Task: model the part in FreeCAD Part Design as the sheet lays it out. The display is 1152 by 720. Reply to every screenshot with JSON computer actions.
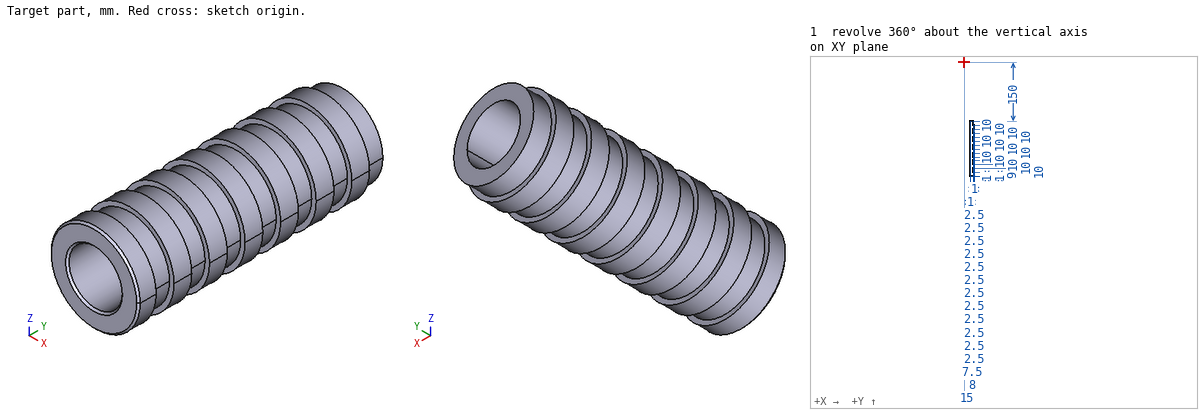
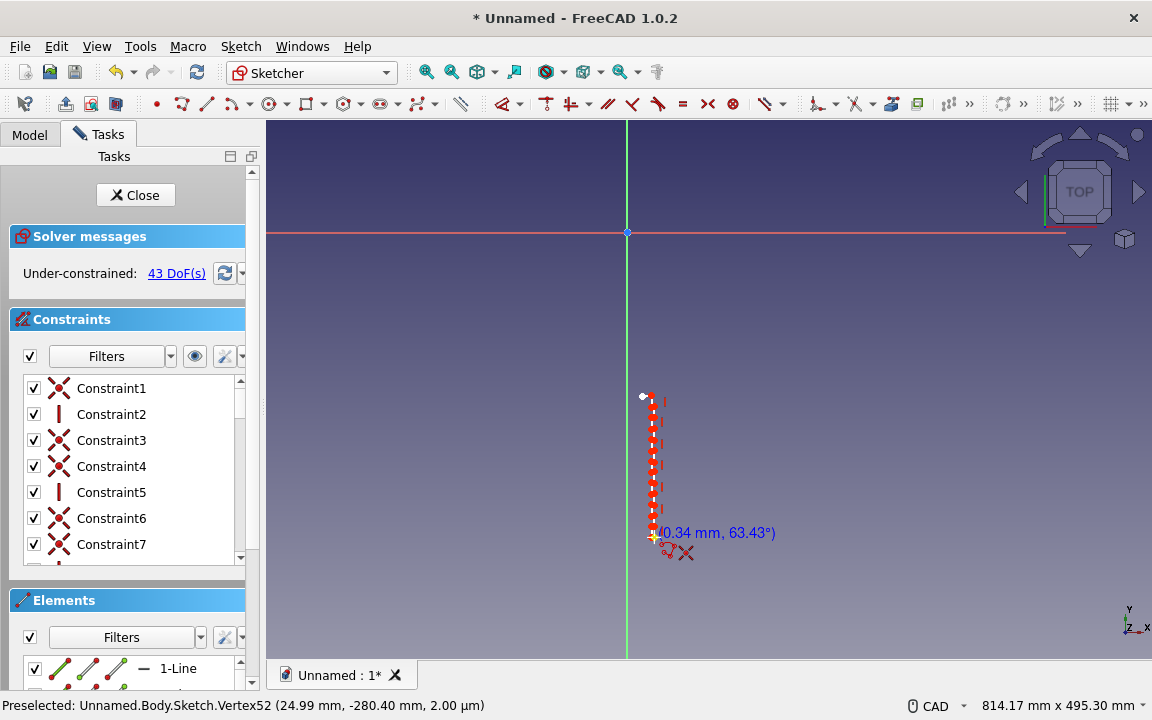
{"action": "scroll", "coordinate": [654, 547], "scroll_direction": "up", "scroll_amount": 3}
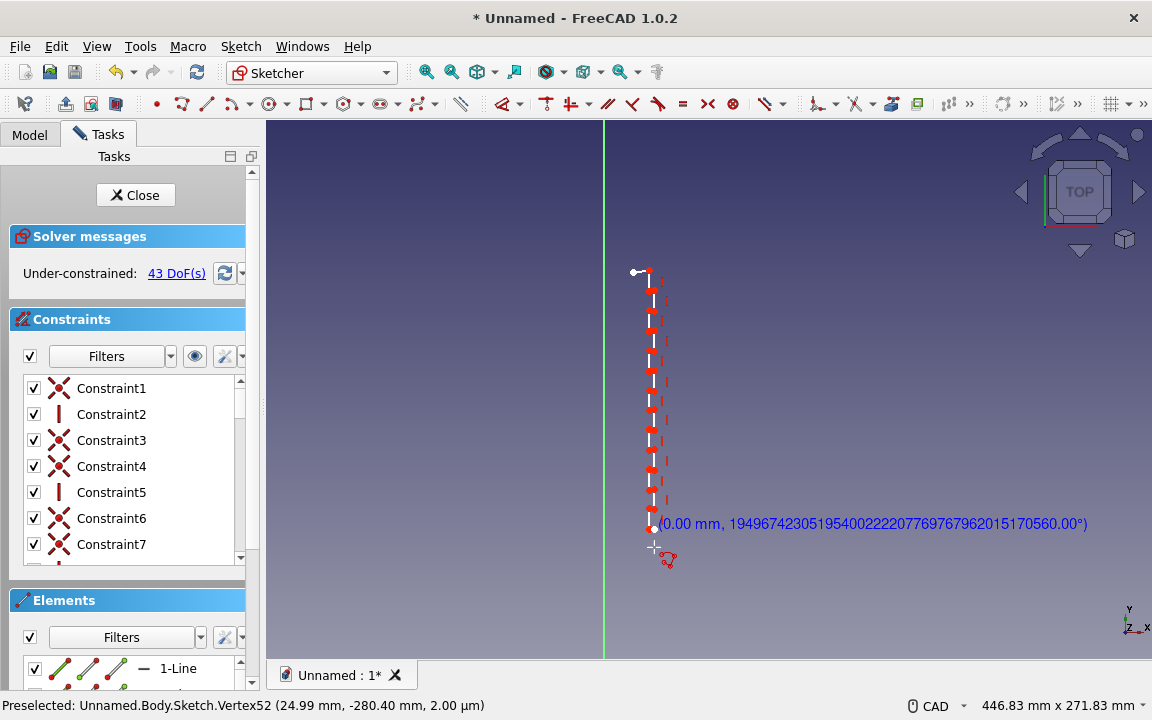
{"action": "left_click", "coordinate": [654, 546]}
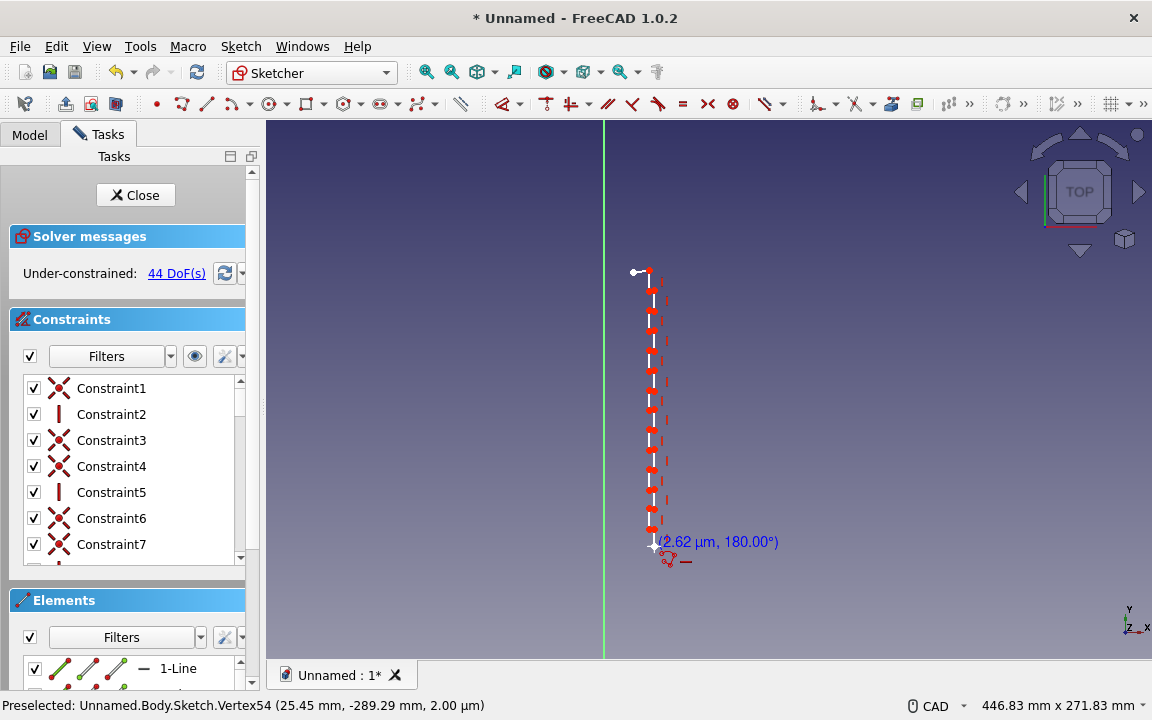
{"action": "scroll", "coordinate": [652, 548], "scroll_direction": "up", "scroll_amount": 9}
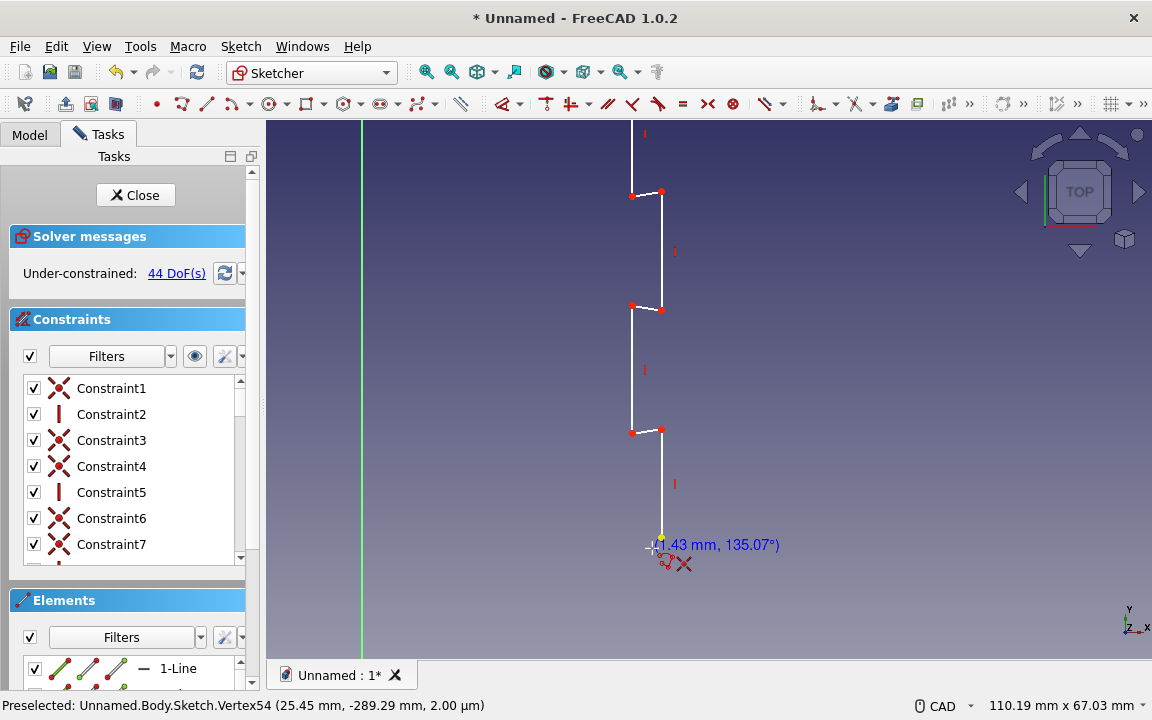
{"action": "left_click", "coordinate": [650, 546]}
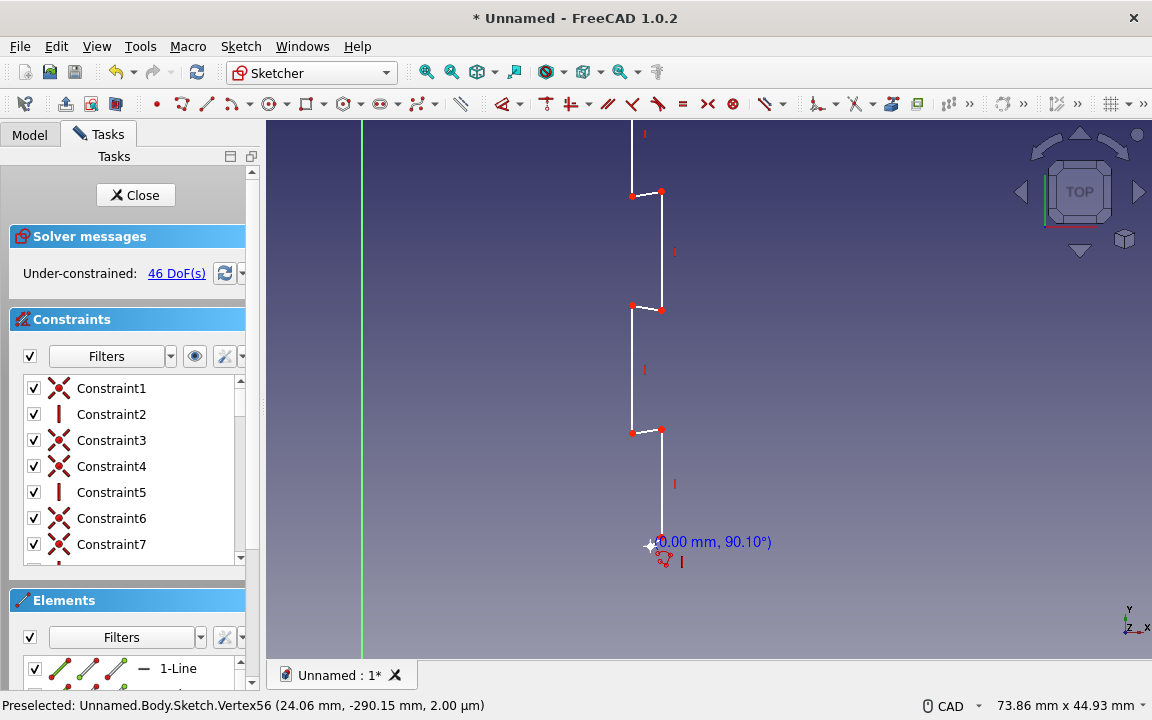
{"action": "scroll", "coordinate": [653, 547], "scroll_direction": "down", "scroll_amount": 12}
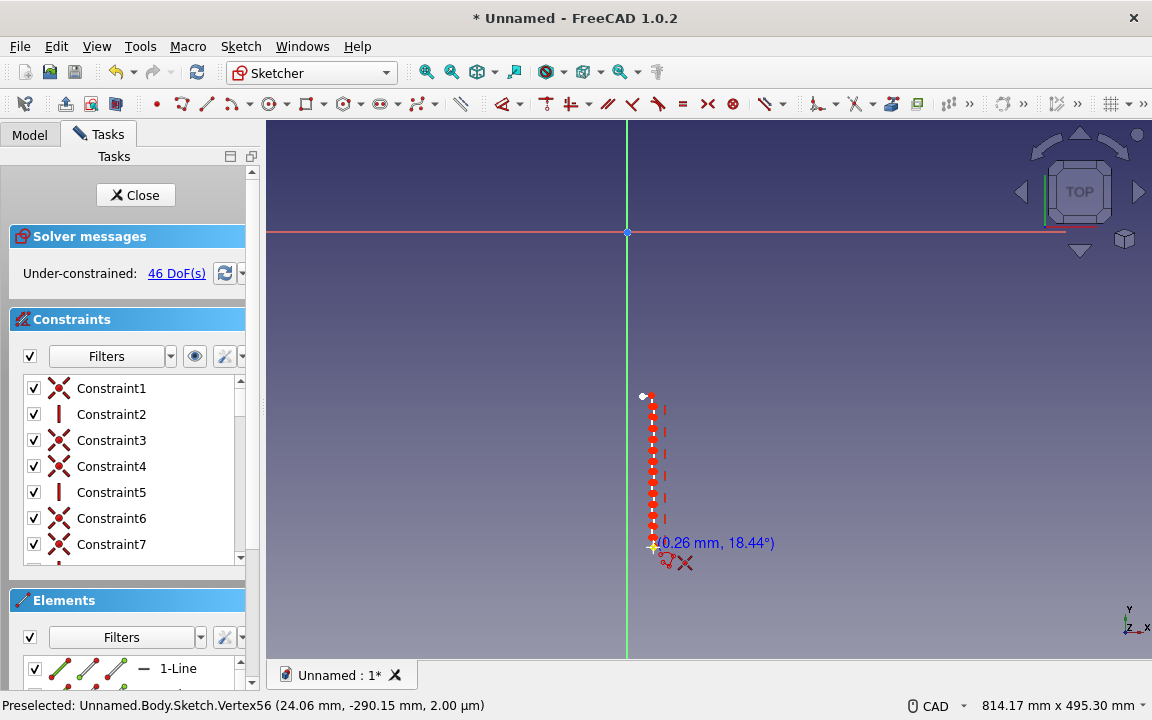
{"action": "scroll", "coordinate": [644, 548], "scroll_direction": "up", "scroll_amount": 4}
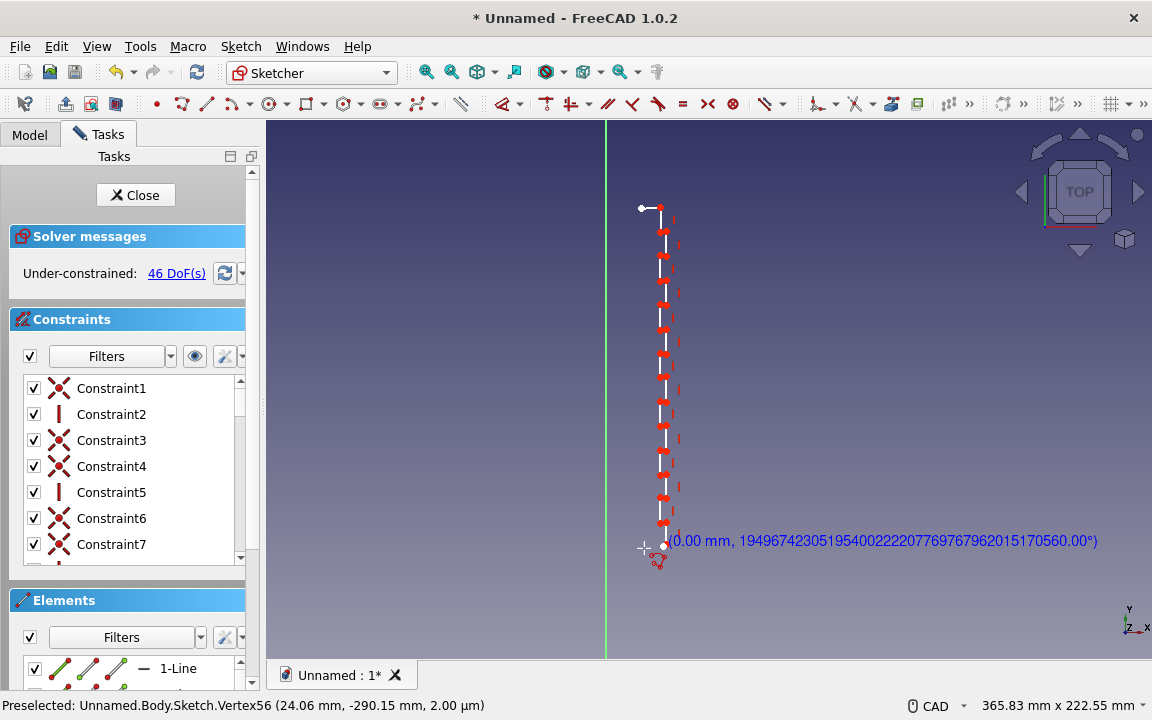
{"action": "left_click", "coordinate": [644, 546]}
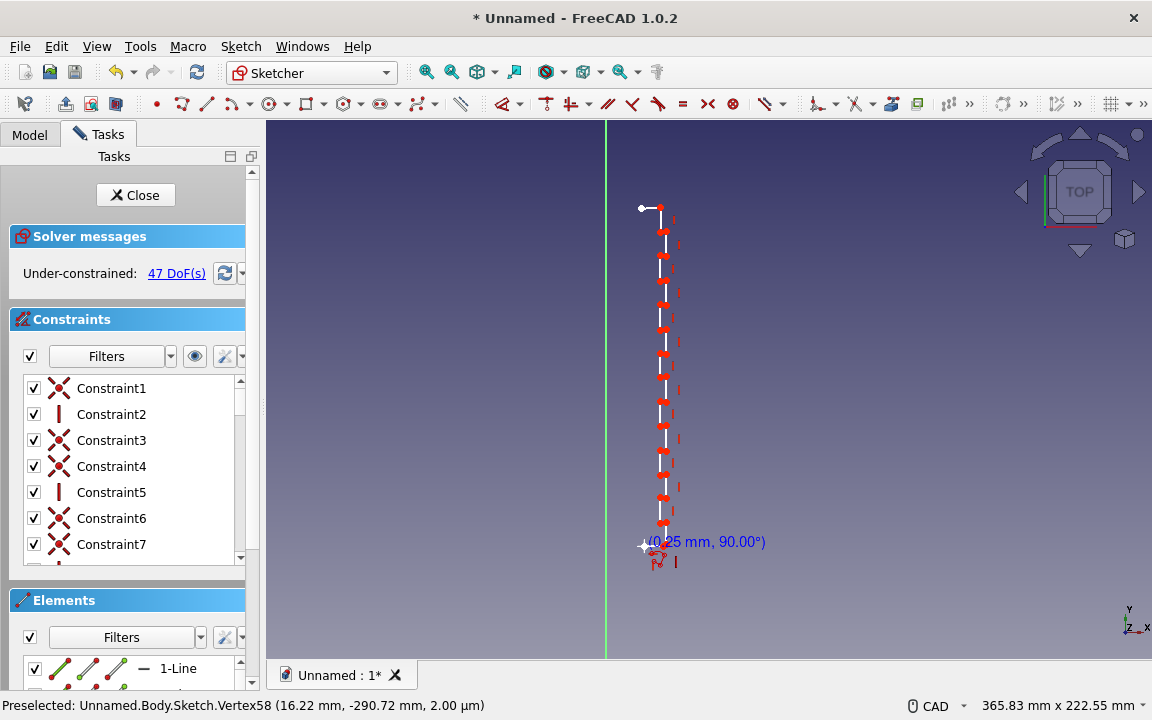
{"action": "scroll", "coordinate": [642, 544], "scroll_direction": "up", "scroll_amount": 8}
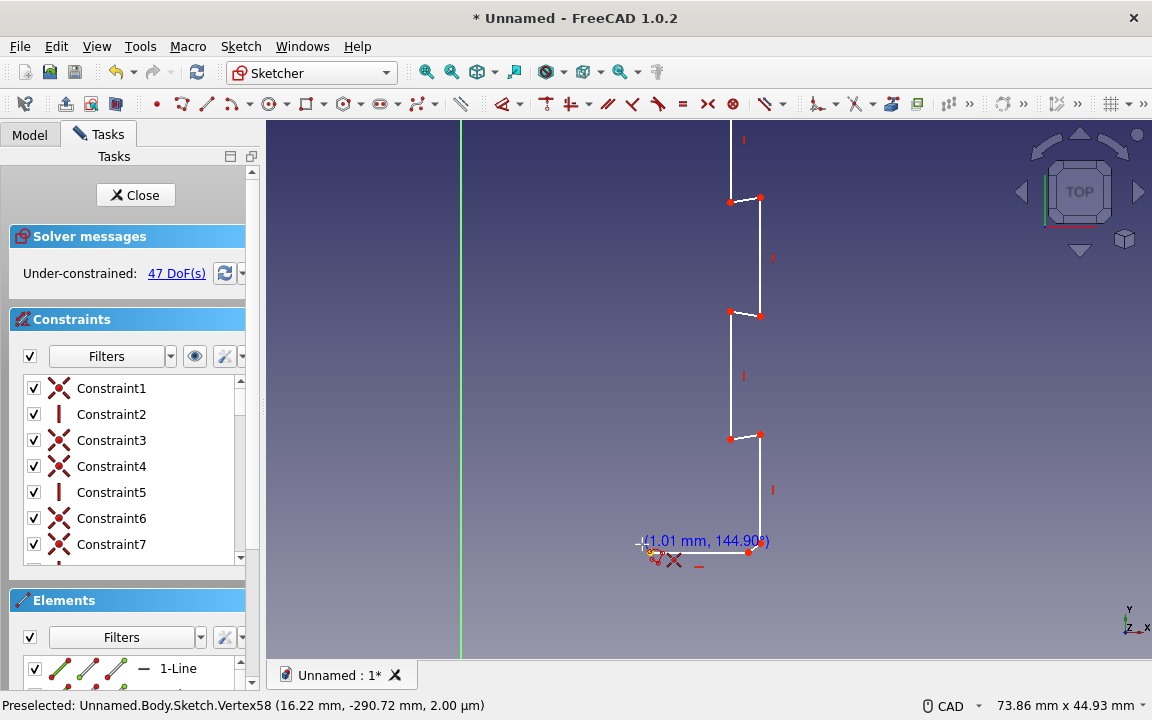
{"action": "left_click", "coordinate": [640, 540]}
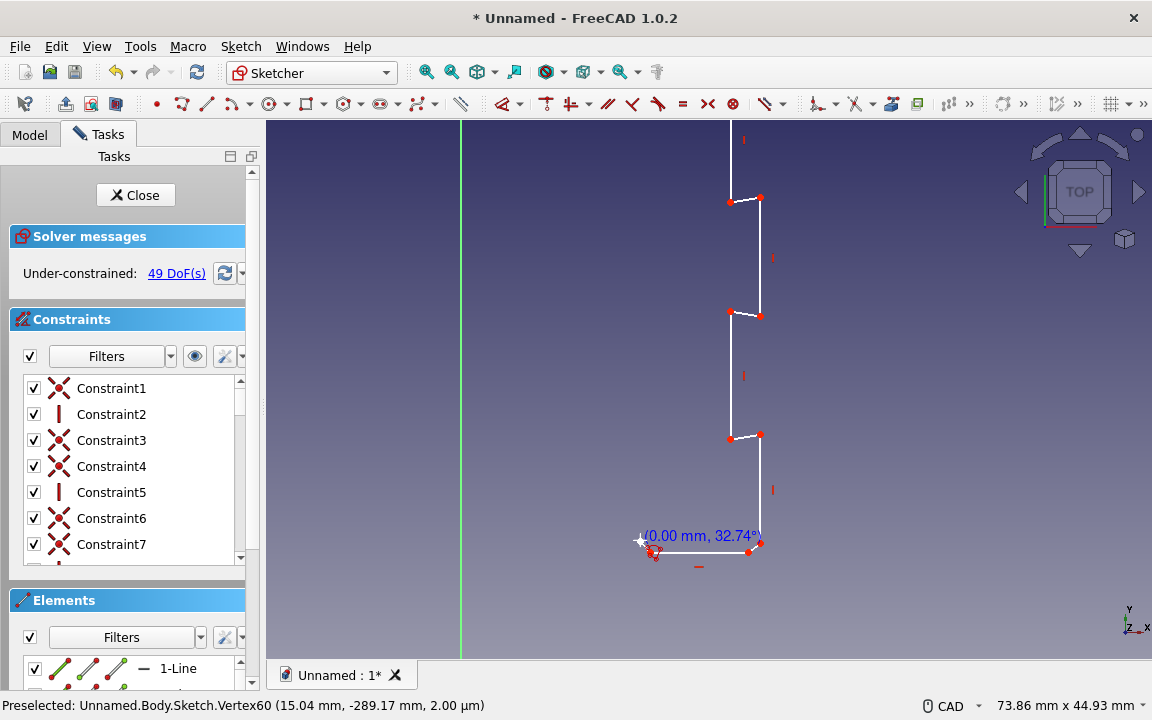
{"action": "scroll", "coordinate": [643, 547], "scroll_direction": "down", "scroll_amount": 12}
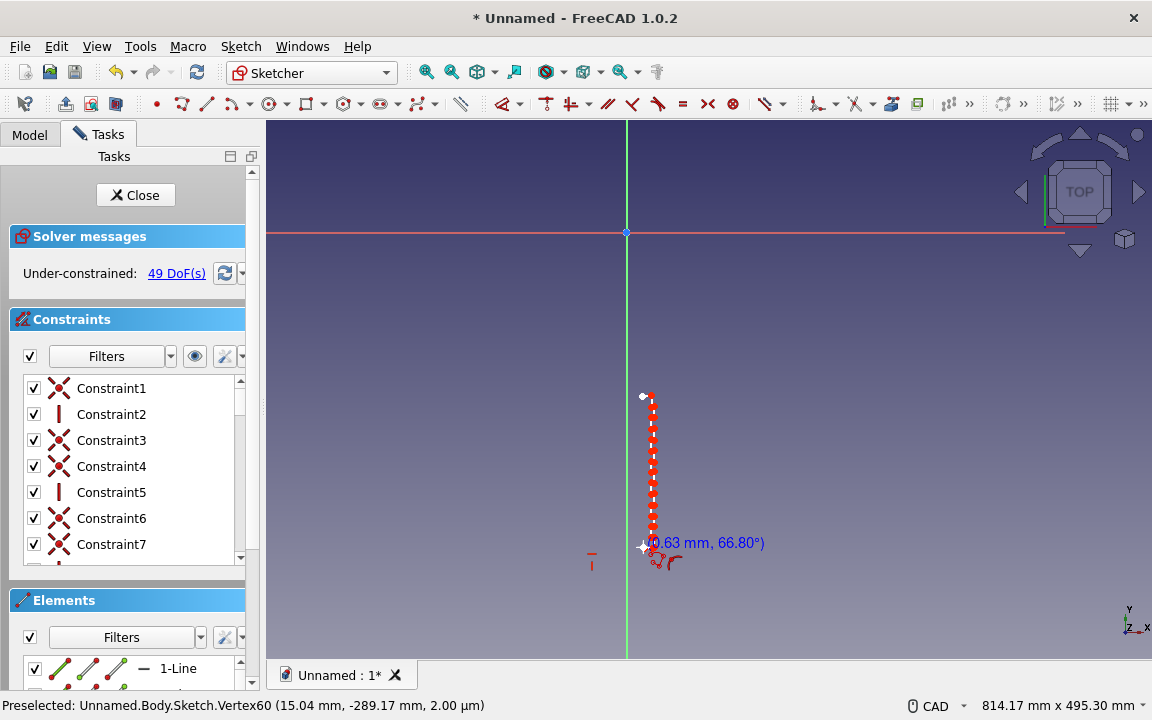
{"action": "scroll", "coordinate": [643, 396], "scroll_direction": "up", "scroll_amount": 7}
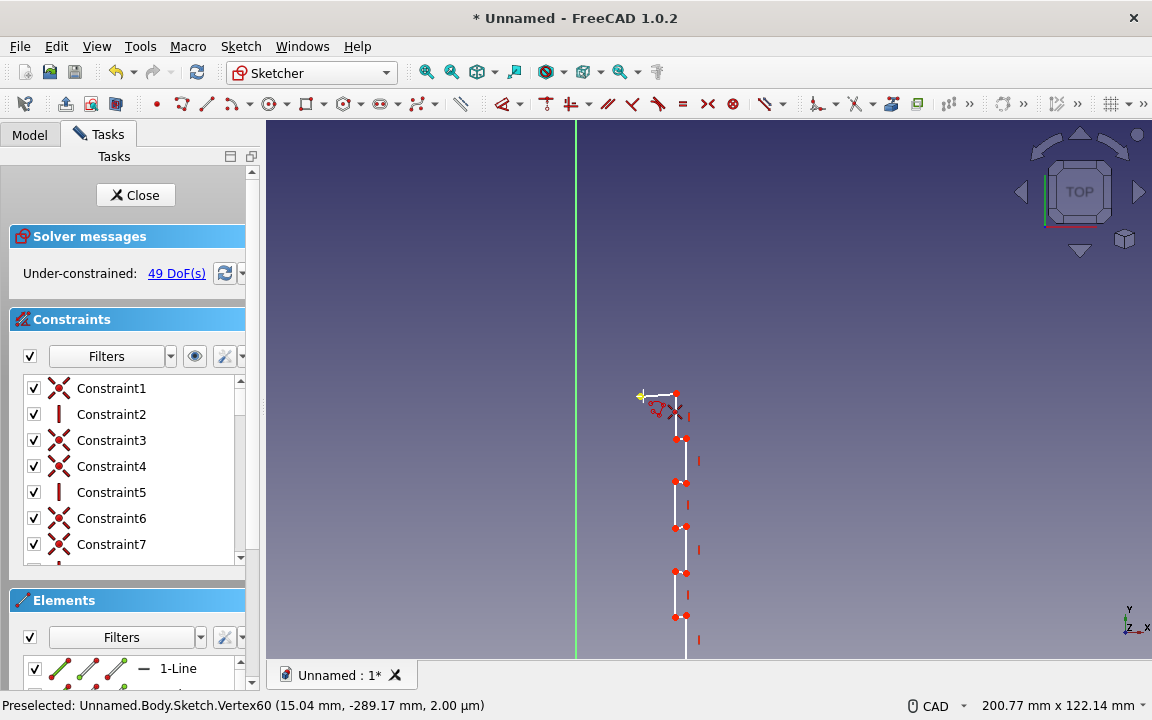
{"action": "left_click", "coordinate": [641, 397]}
{"action": "key", "text": "Escape"}
{"action": "key", "text": "Escape"}